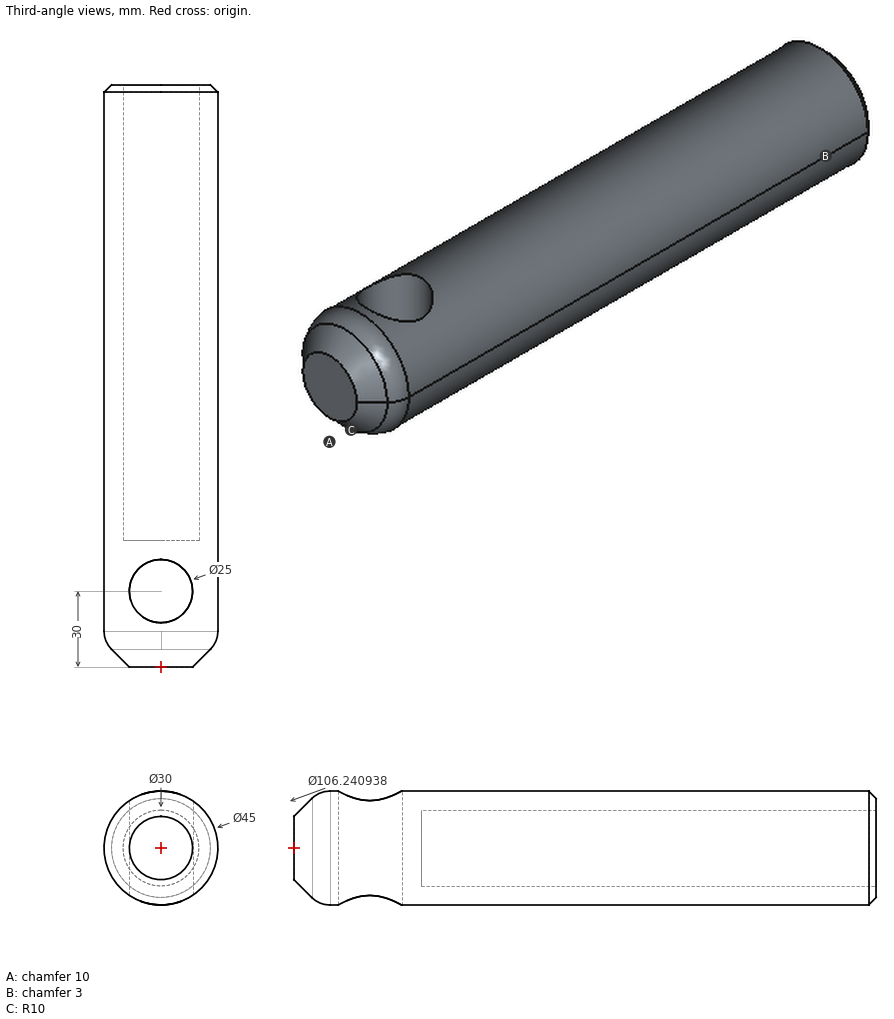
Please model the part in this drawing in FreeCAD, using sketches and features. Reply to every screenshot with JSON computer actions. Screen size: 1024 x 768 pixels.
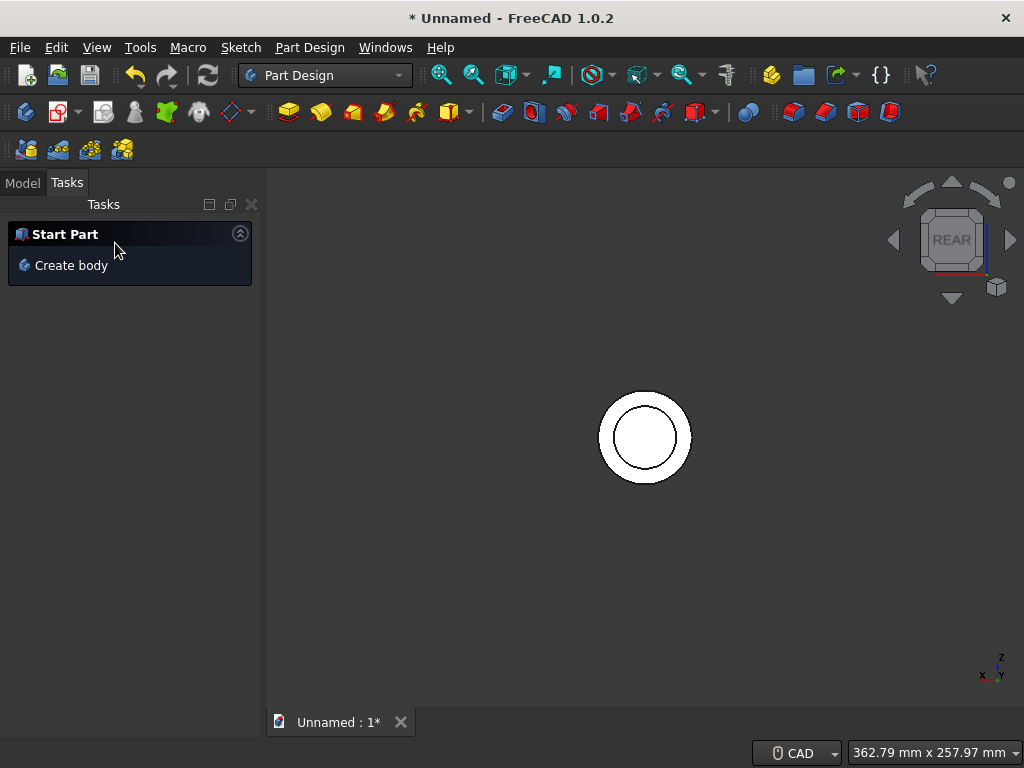
{"action": "left_click", "coordinate": [442, 76]}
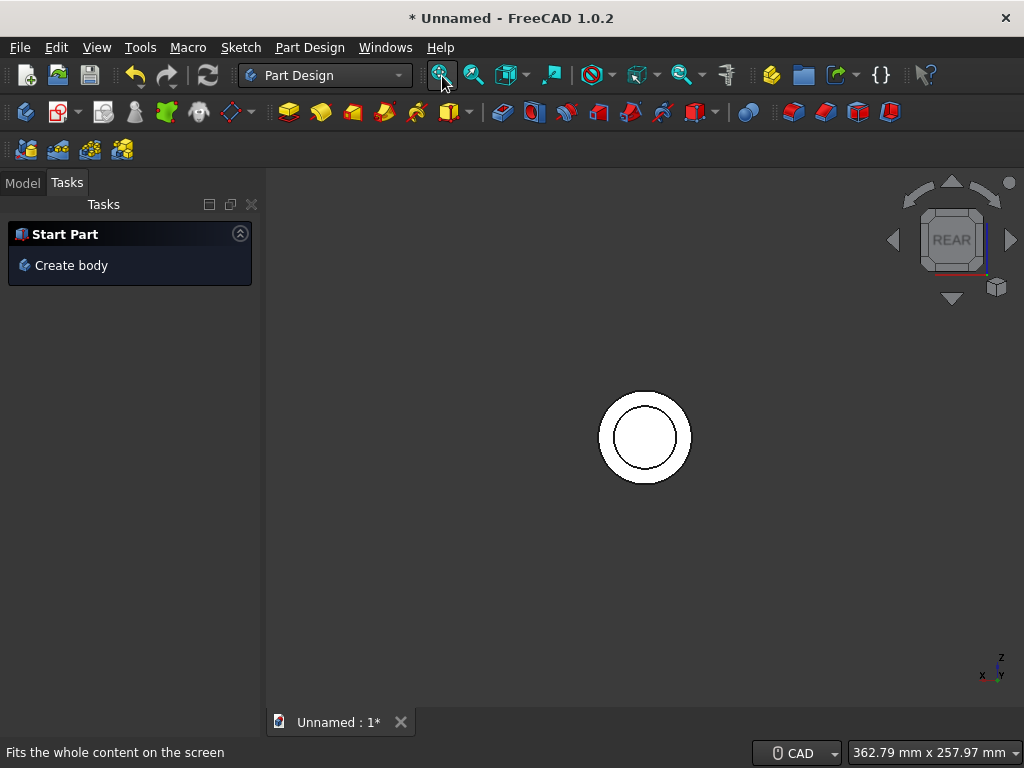
{"action": "left_click", "coordinate": [58, 112]}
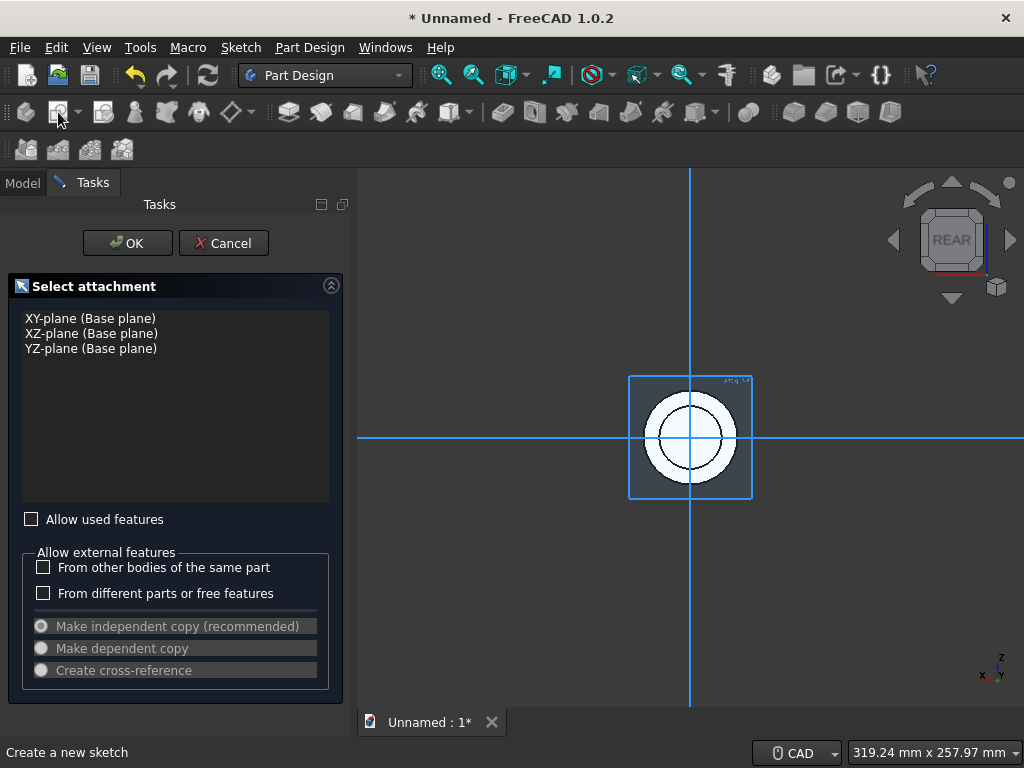
{"action": "left_click", "coordinate": [82, 318]}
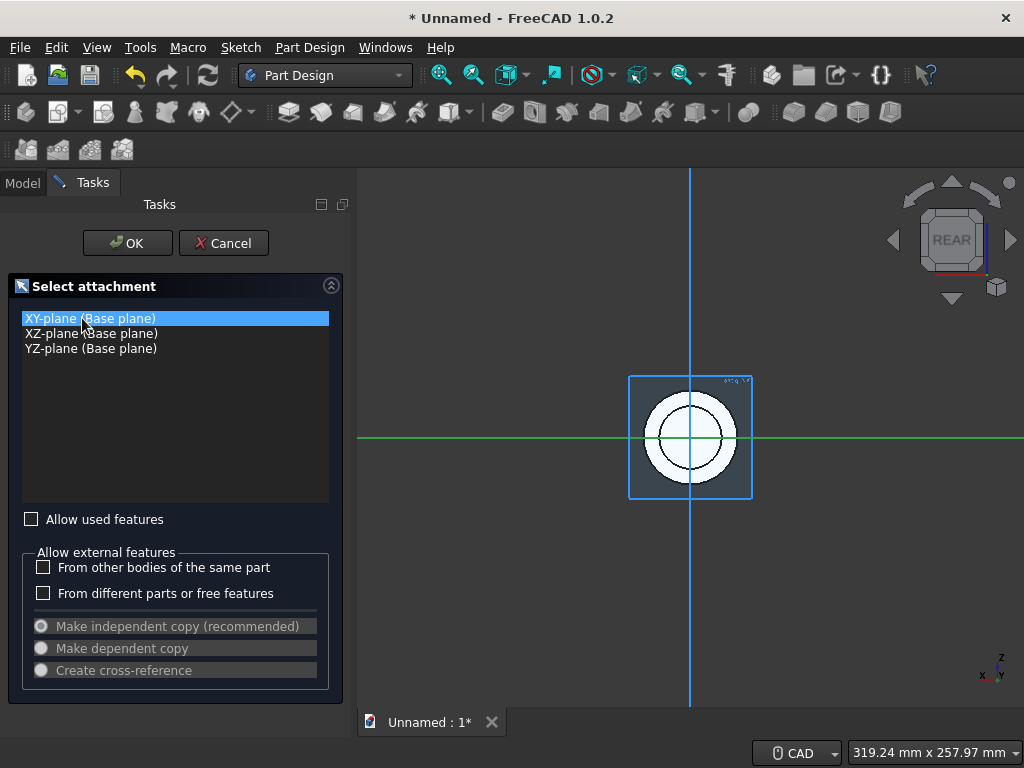
{"action": "left_click", "coordinate": [128, 243]}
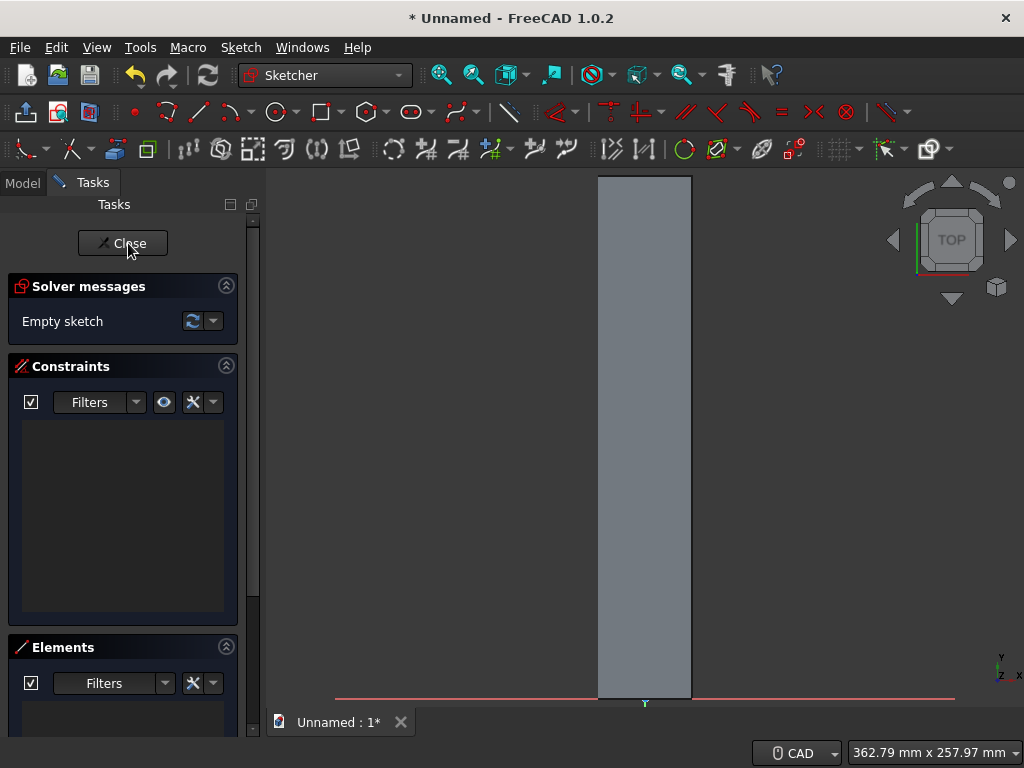
{"action": "key", "text": "q s"}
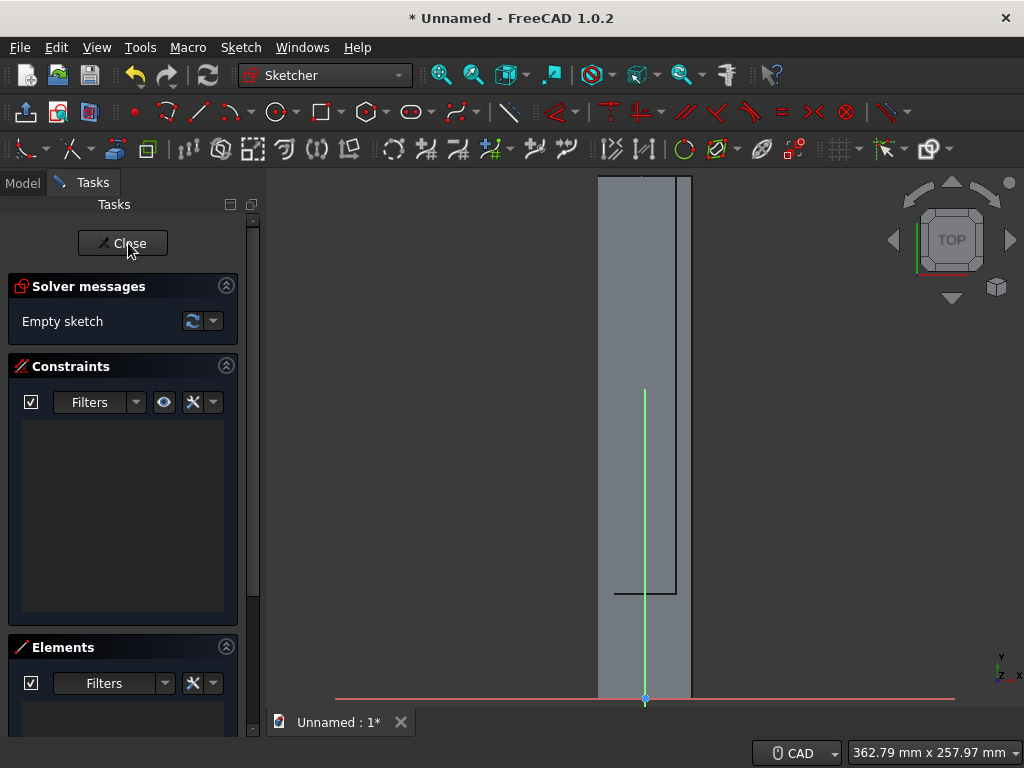
{"action": "scroll", "coordinate": [576, 438], "scroll_direction": "down", "scroll_amount": 5}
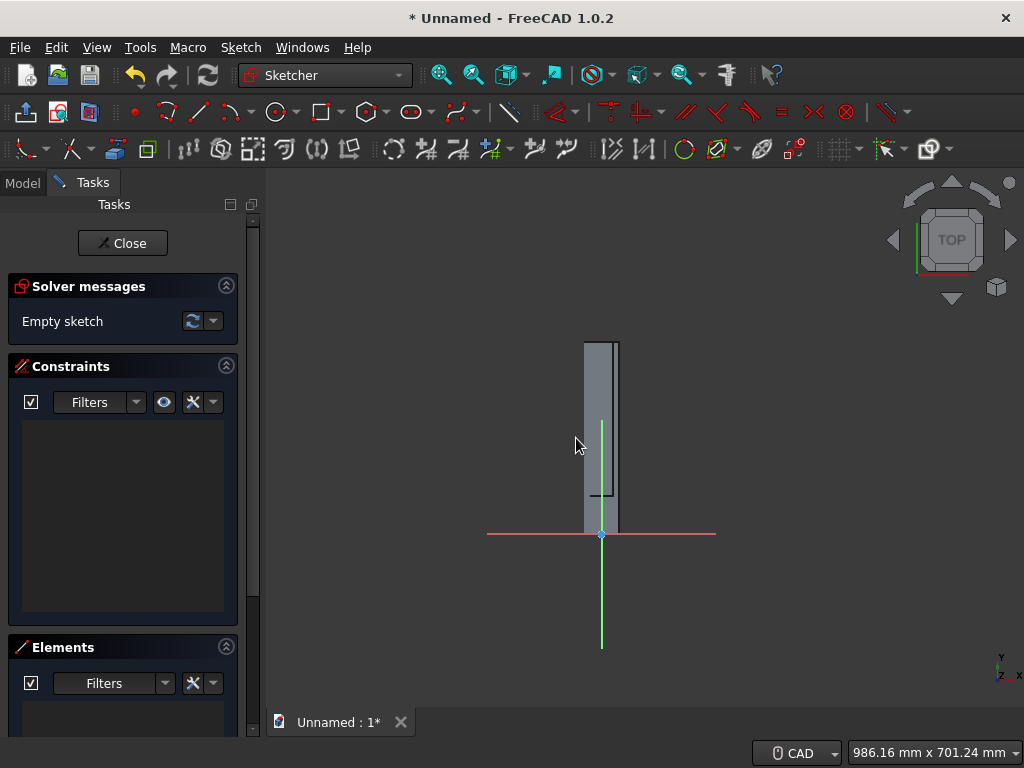
{"action": "scroll", "coordinate": [604, 526], "scroll_direction": "up", "scroll_amount": 12}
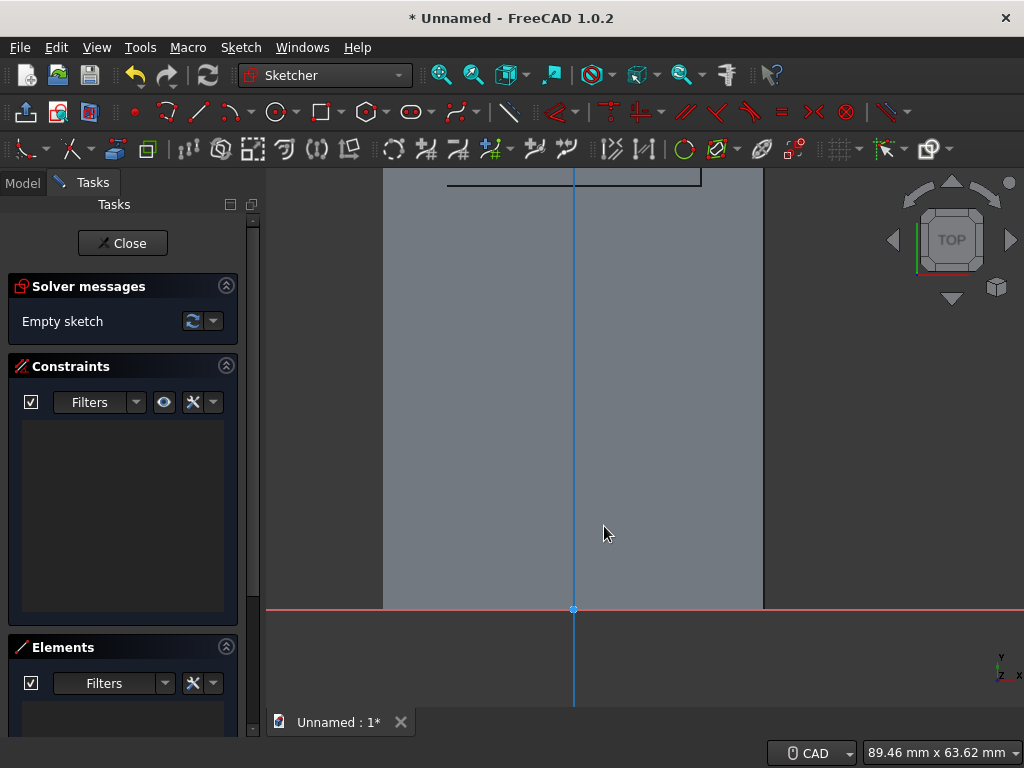
{"action": "key", "text": "g c"}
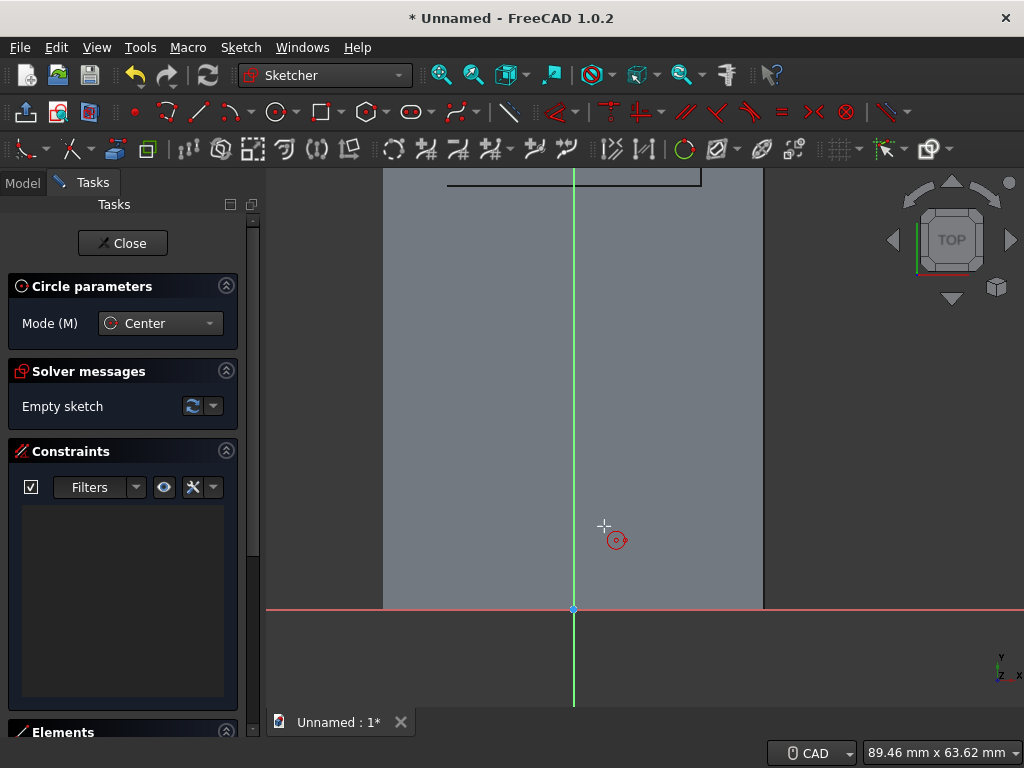
{"action": "left_click", "coordinate": [574, 356]}
{"action": "mouse_move", "coordinate": [648, 281]}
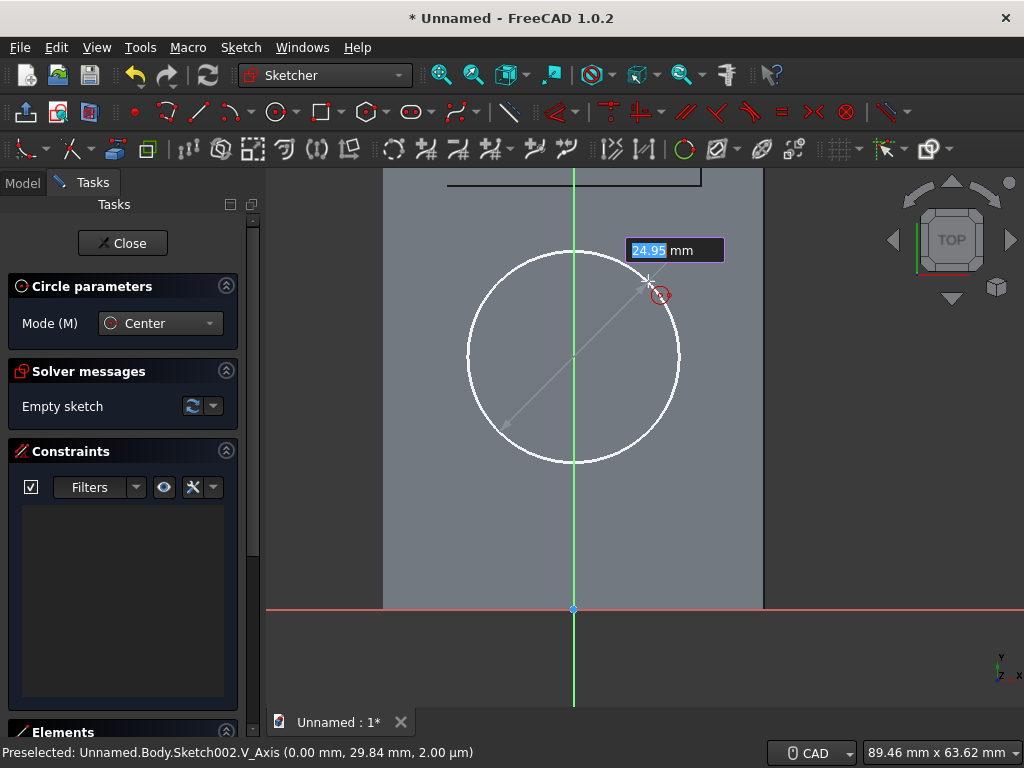
{"action": "type", "text": "25"}
{"action": "key", "text": "Return"}
{"action": "key", "text": "Escape"}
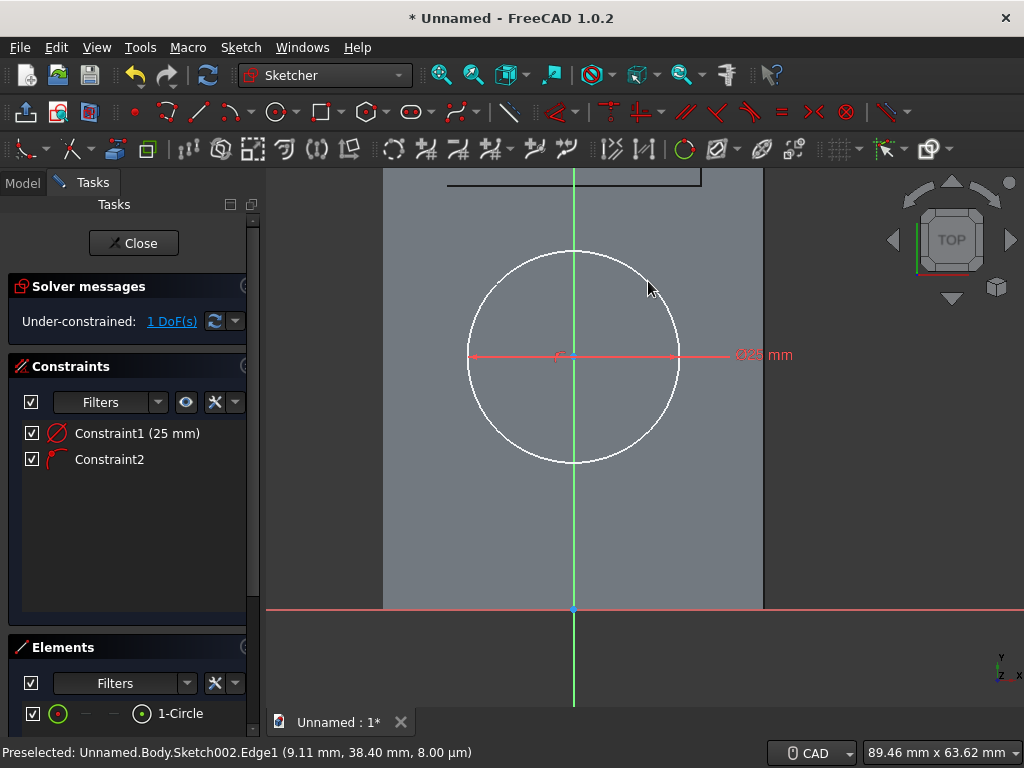
{"action": "left_click", "coordinate": [556, 112]}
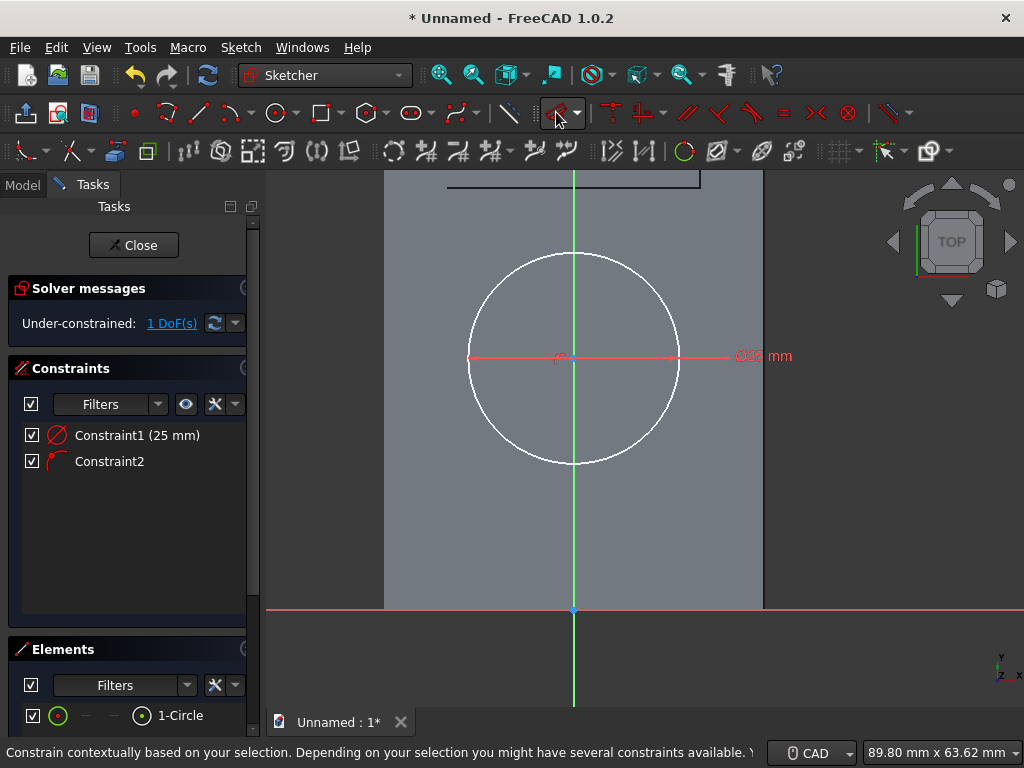
{"action": "left_click", "coordinate": [574, 358]}
{"action": "left_click", "coordinate": [608, 484]}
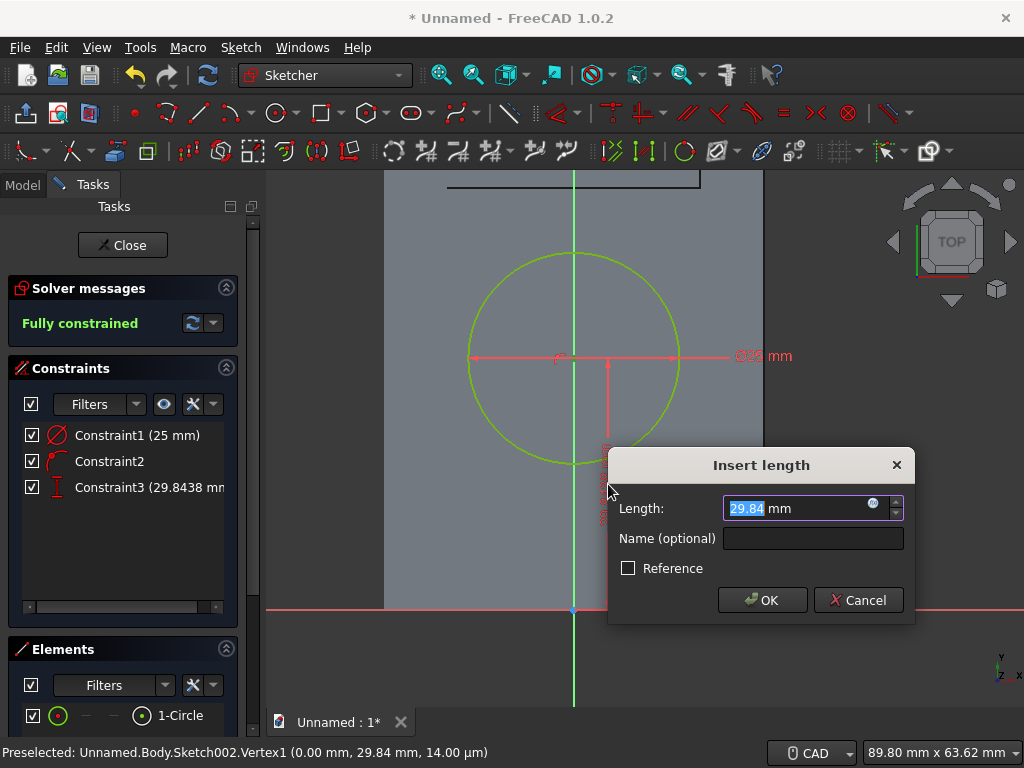
{"action": "type", "text": "30"}
{"action": "key", "text": "Return"}
{"action": "key", "text": "Escape"}